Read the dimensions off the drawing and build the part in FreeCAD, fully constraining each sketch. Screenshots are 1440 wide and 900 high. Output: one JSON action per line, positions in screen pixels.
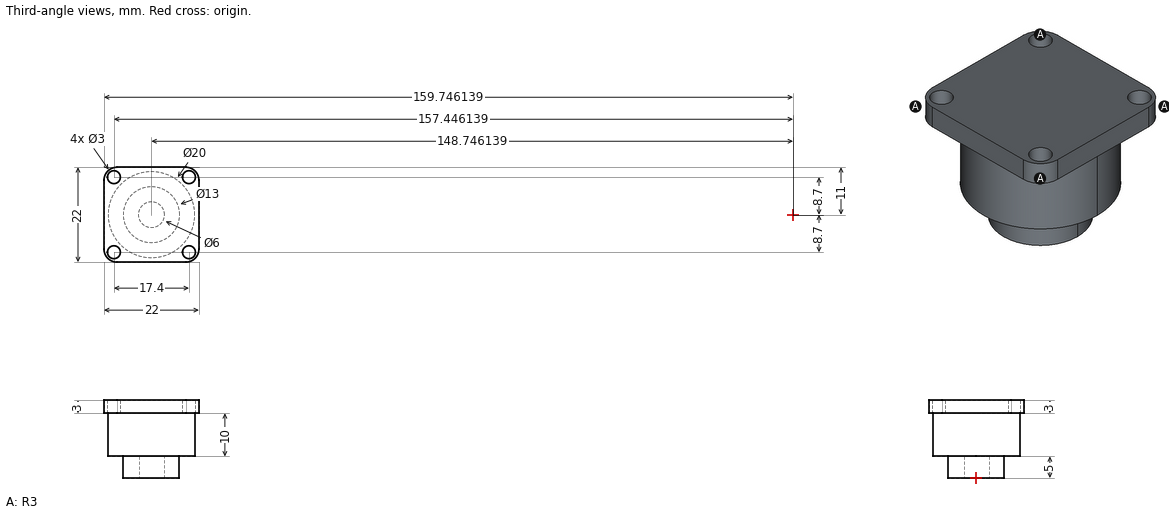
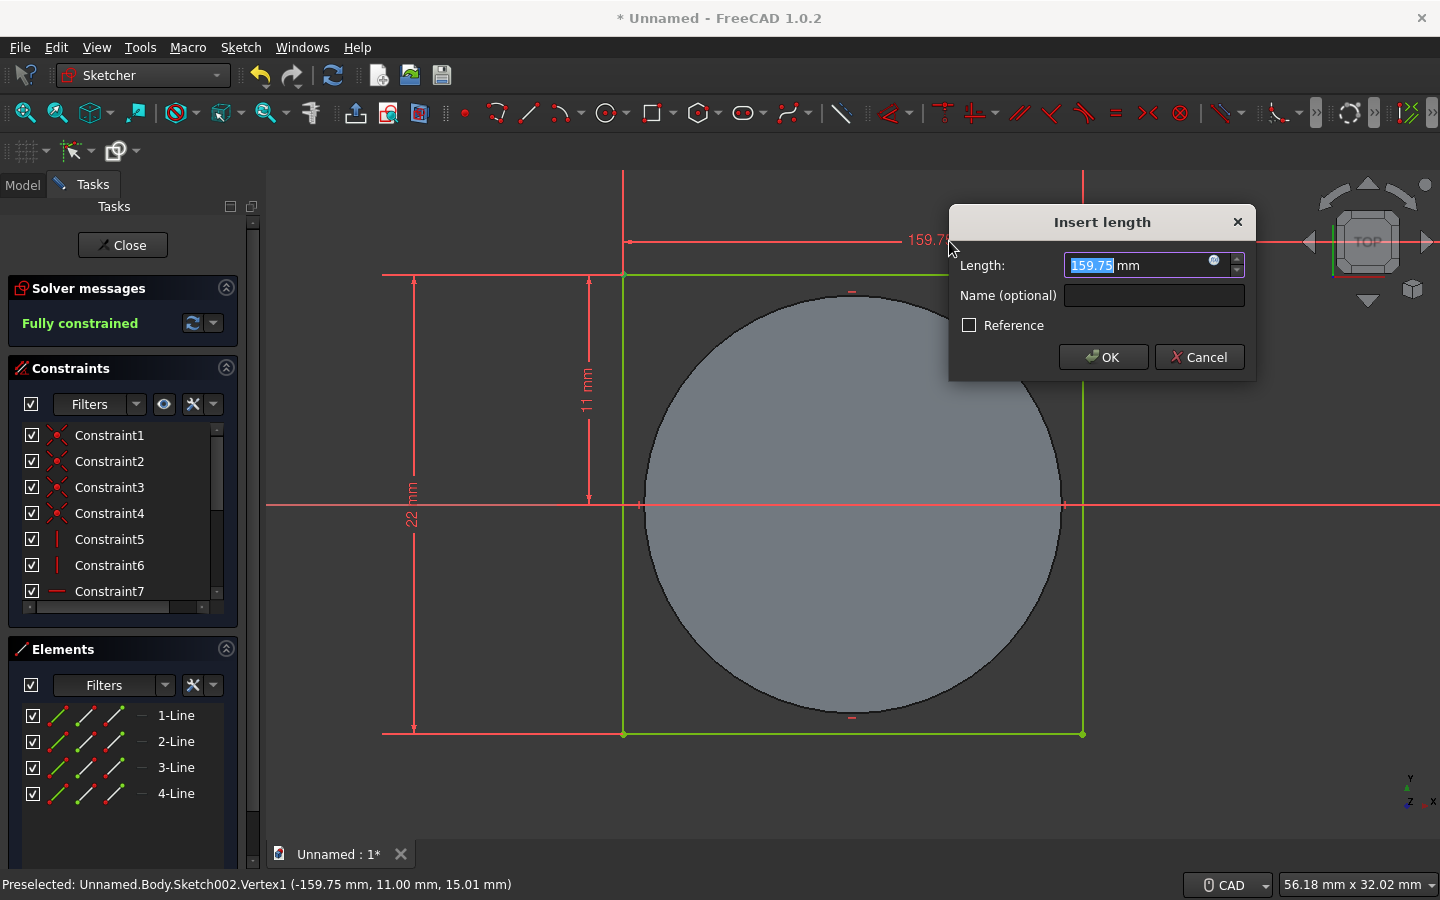
{"action": "type", "text": "159.746139"}
{"action": "key", "text": "Return"}
{"action": "key", "text": "Escape"}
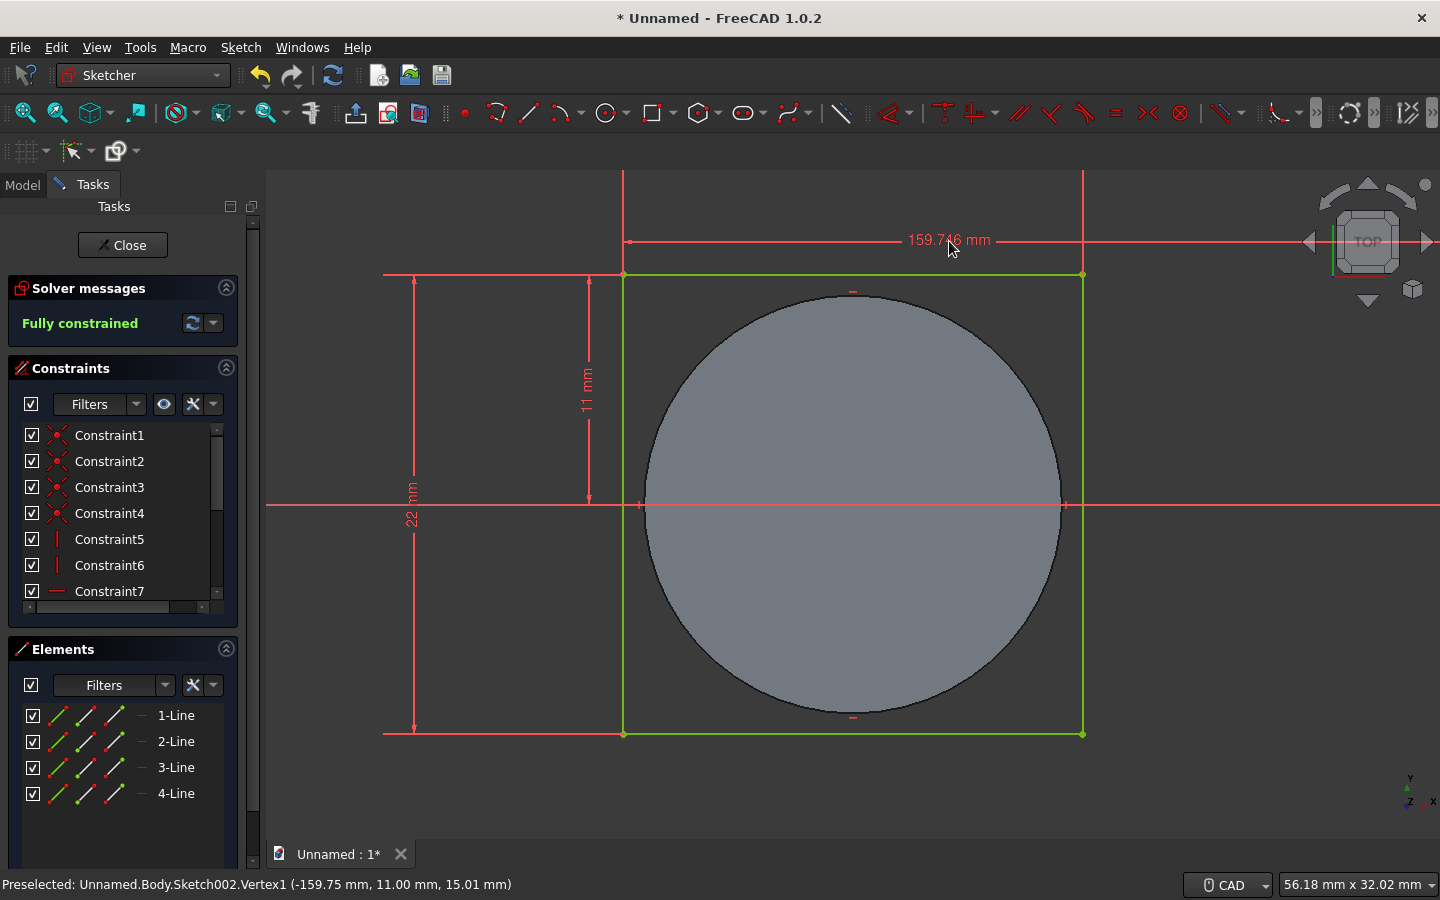
{"action": "left_click", "coordinate": [123, 245]}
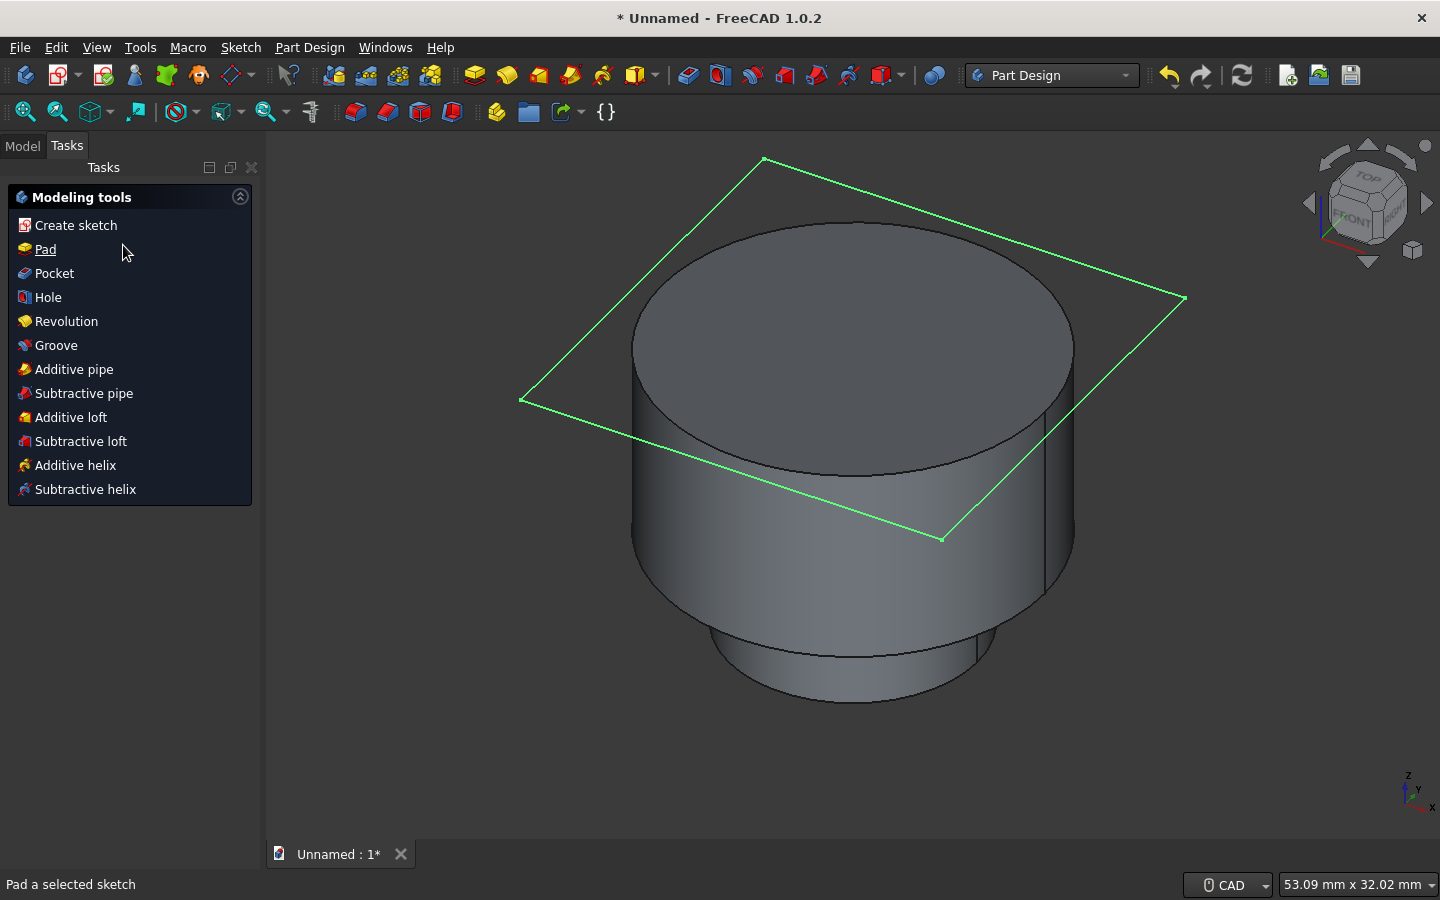
{"action": "left_click", "coordinate": [476, 76]}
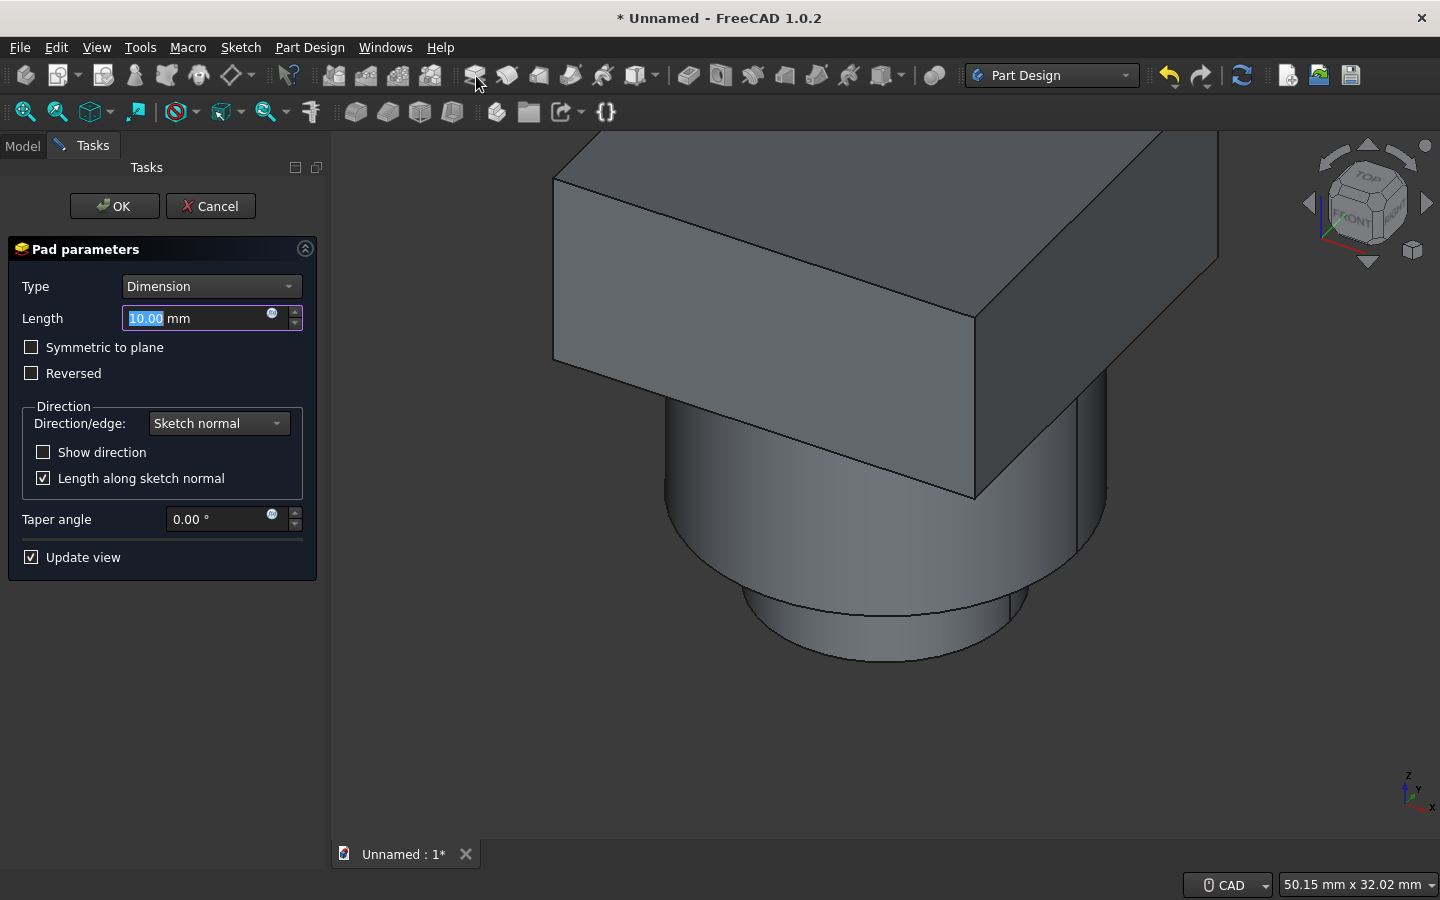
{"action": "type", "text": "3"}
{"action": "key", "text": "Tab"}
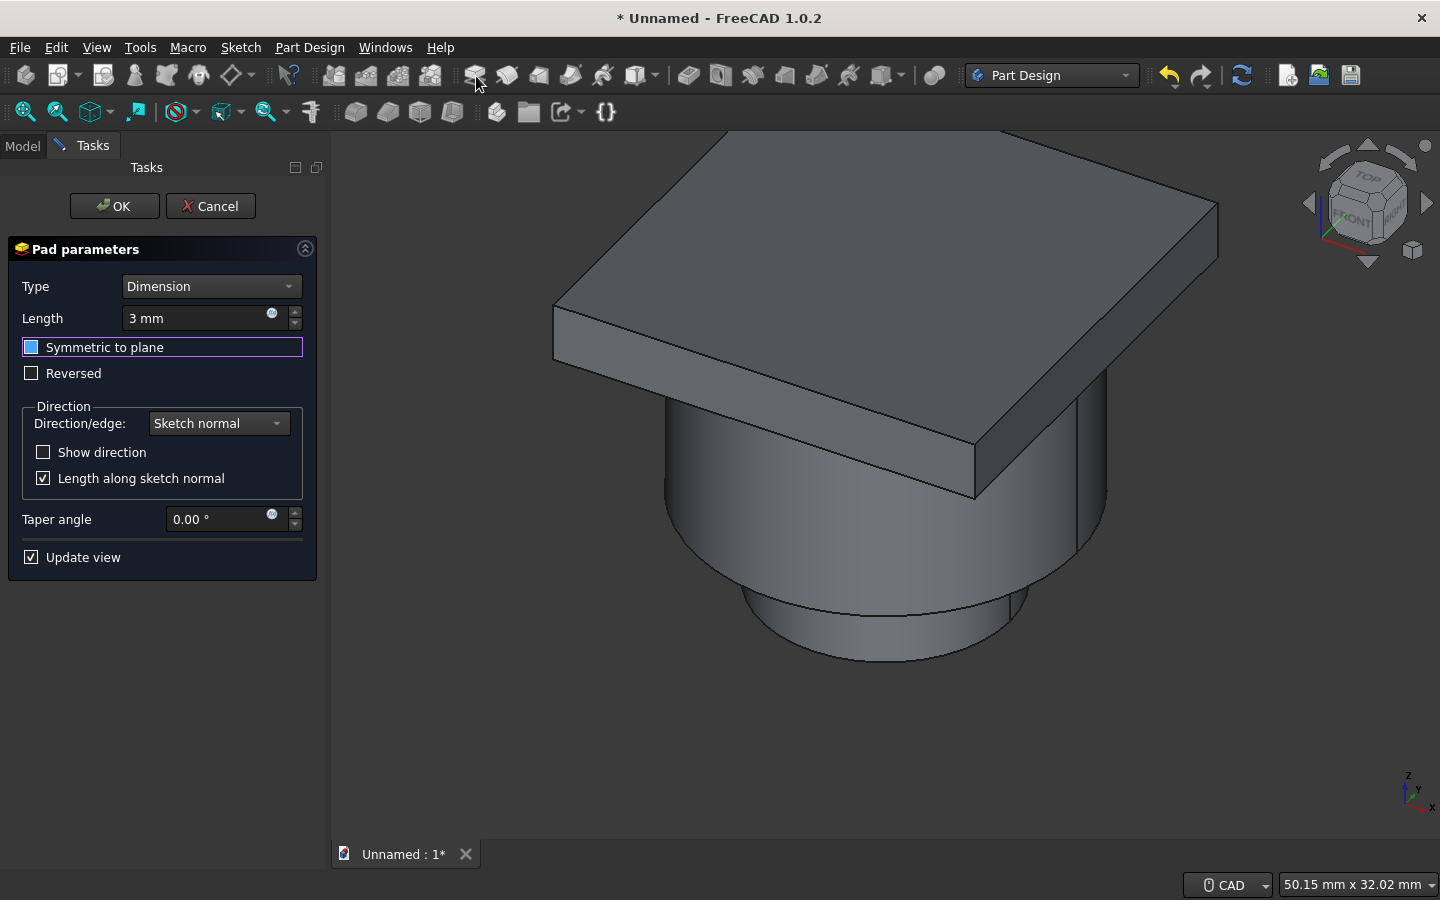
{"action": "left_click", "coordinate": [115, 206]}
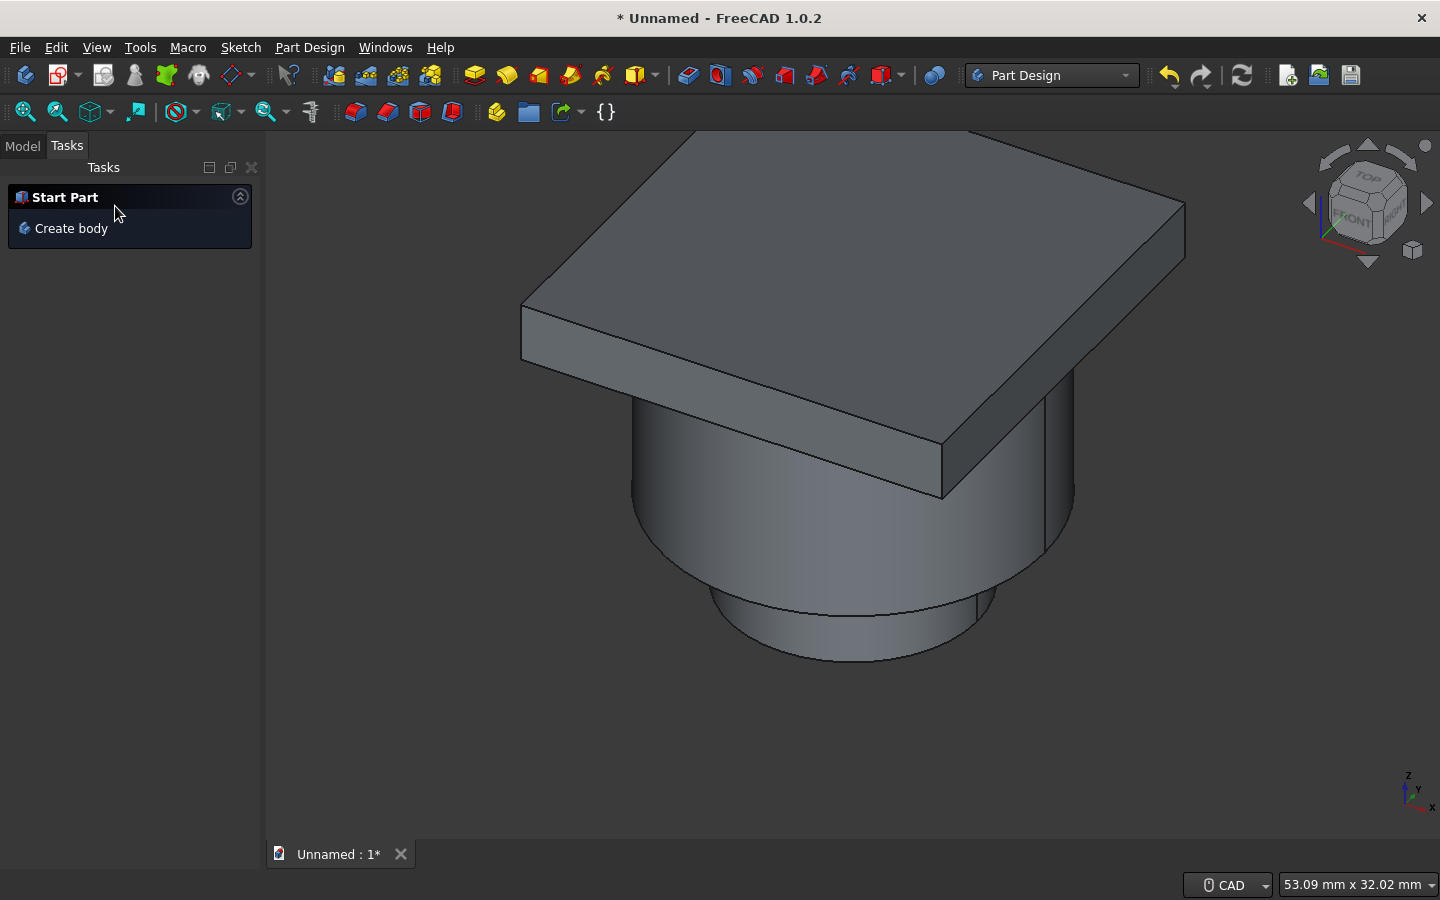
{"action": "left_click", "coordinate": [26, 112]}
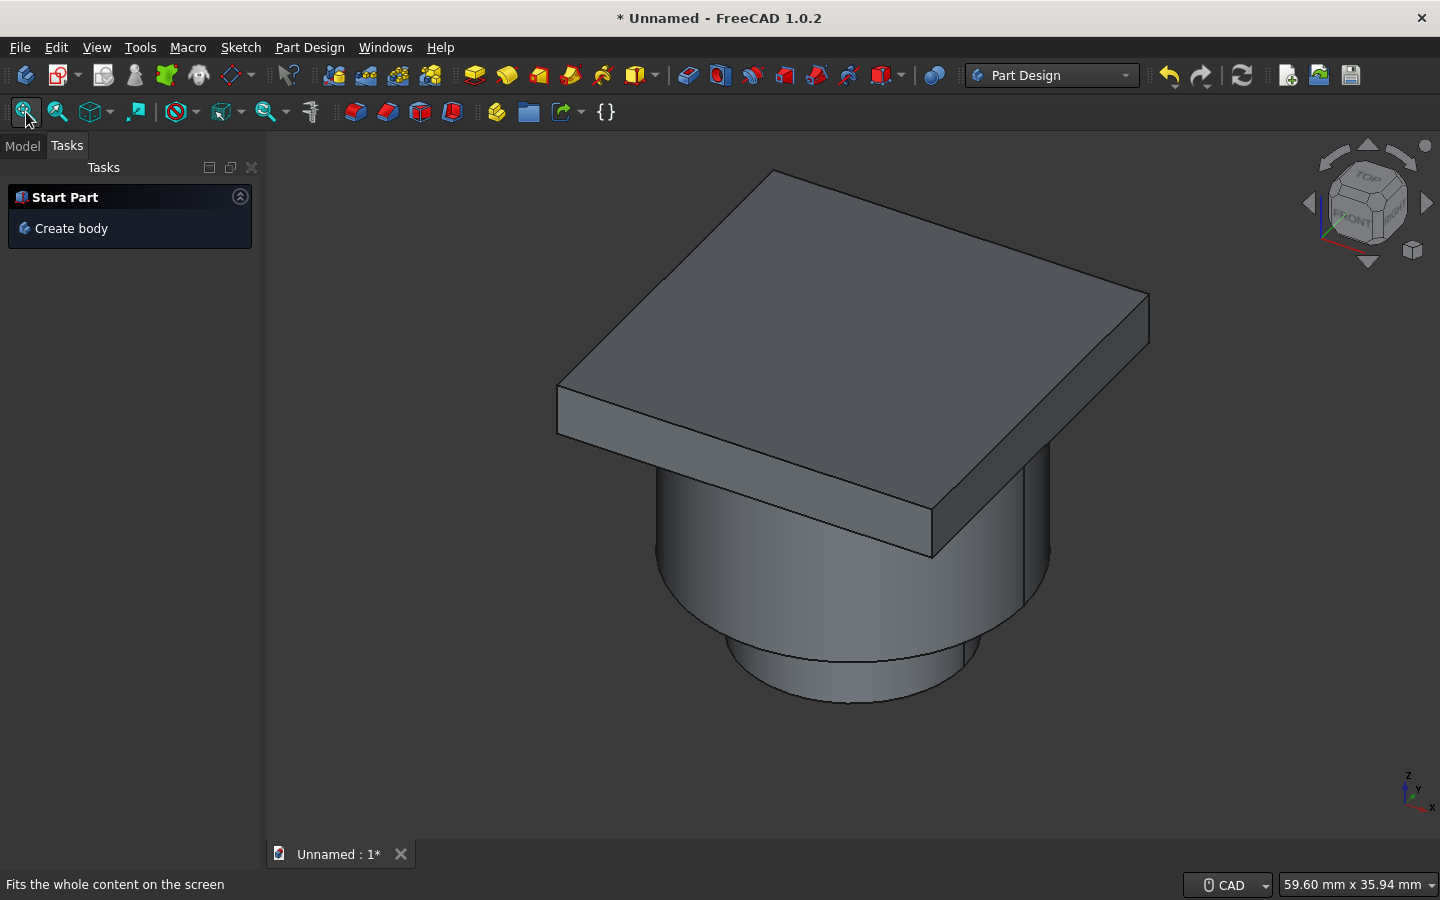
{"action": "left_click", "coordinate": [932, 533]}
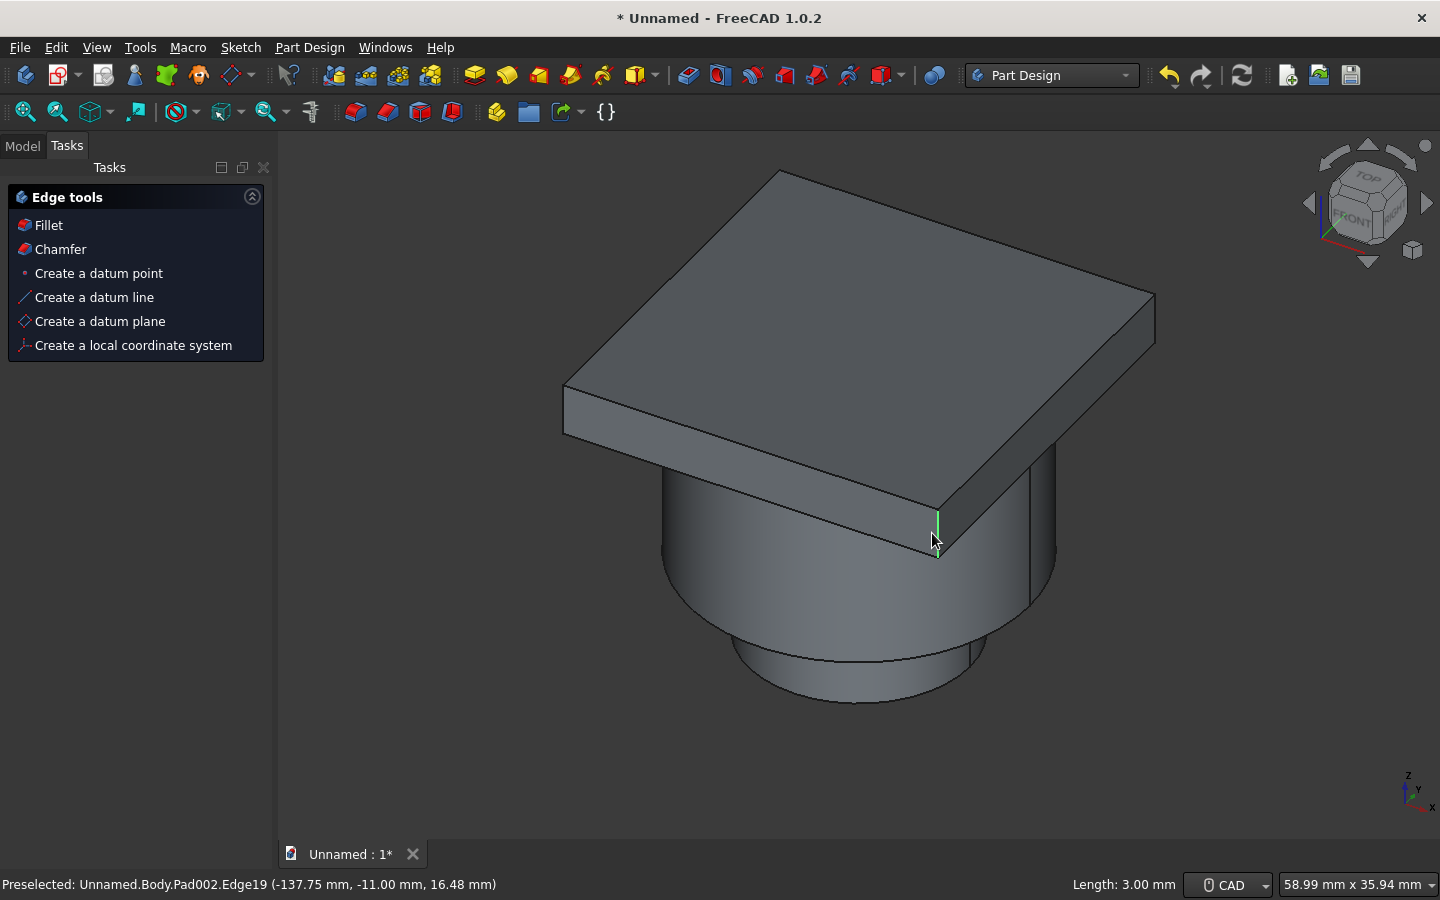
{"action": "key", "text": "0"}